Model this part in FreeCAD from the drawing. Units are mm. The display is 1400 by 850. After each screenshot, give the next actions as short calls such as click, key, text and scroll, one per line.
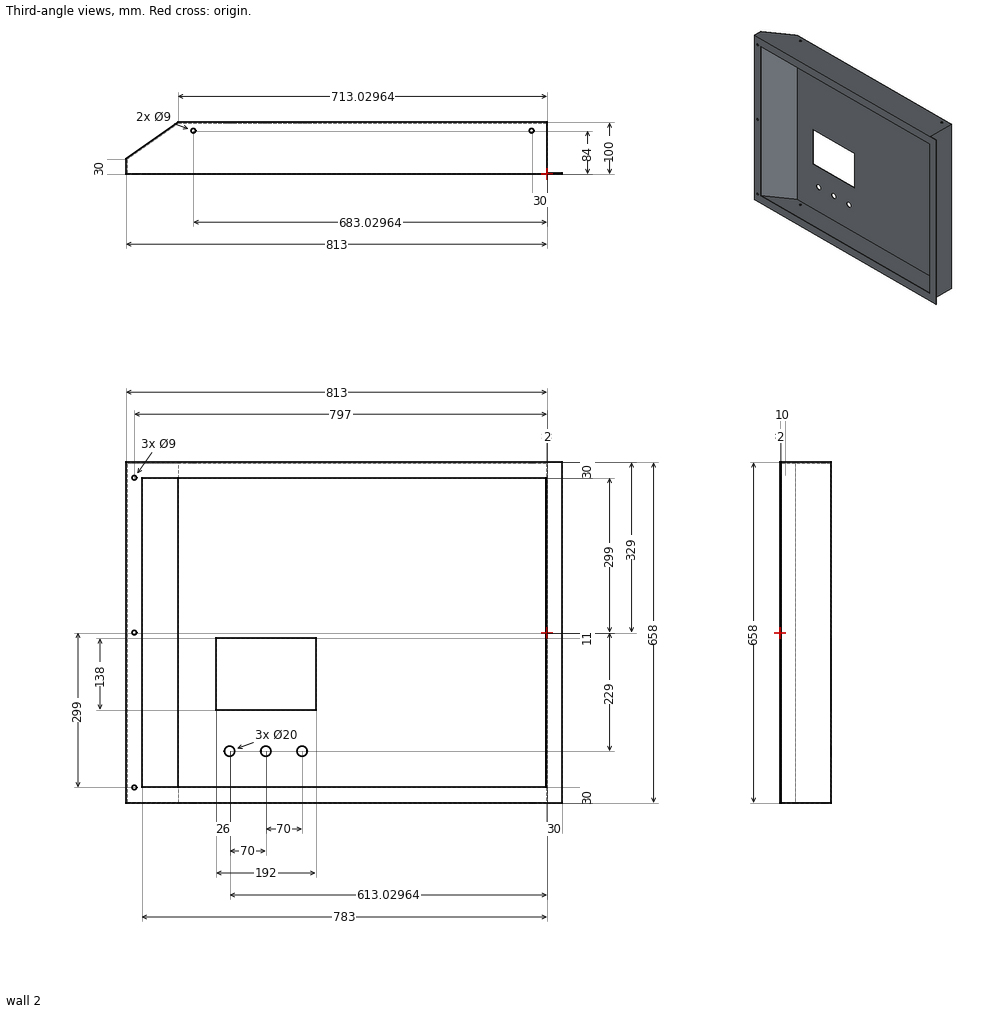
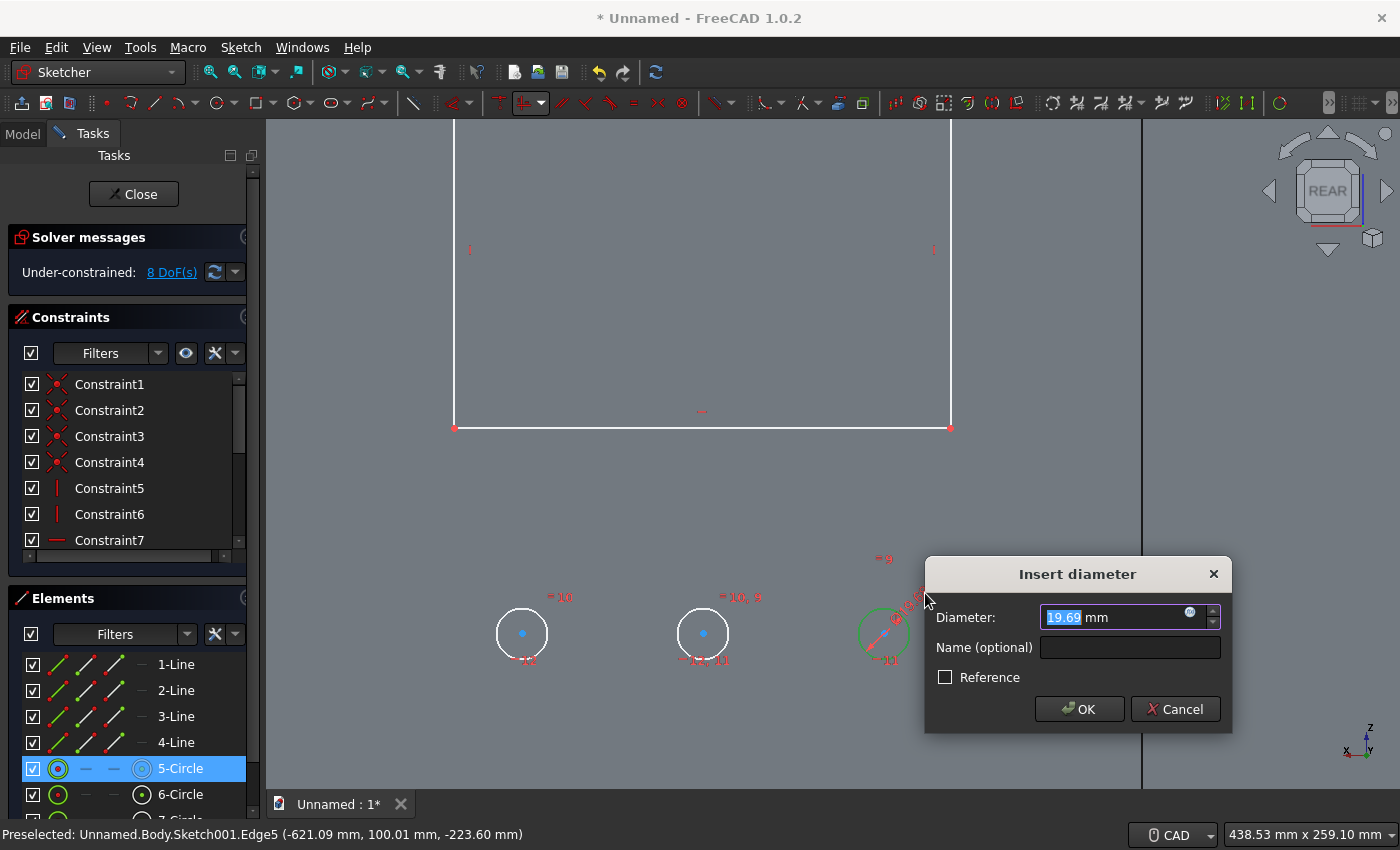
text(20)
key(Return)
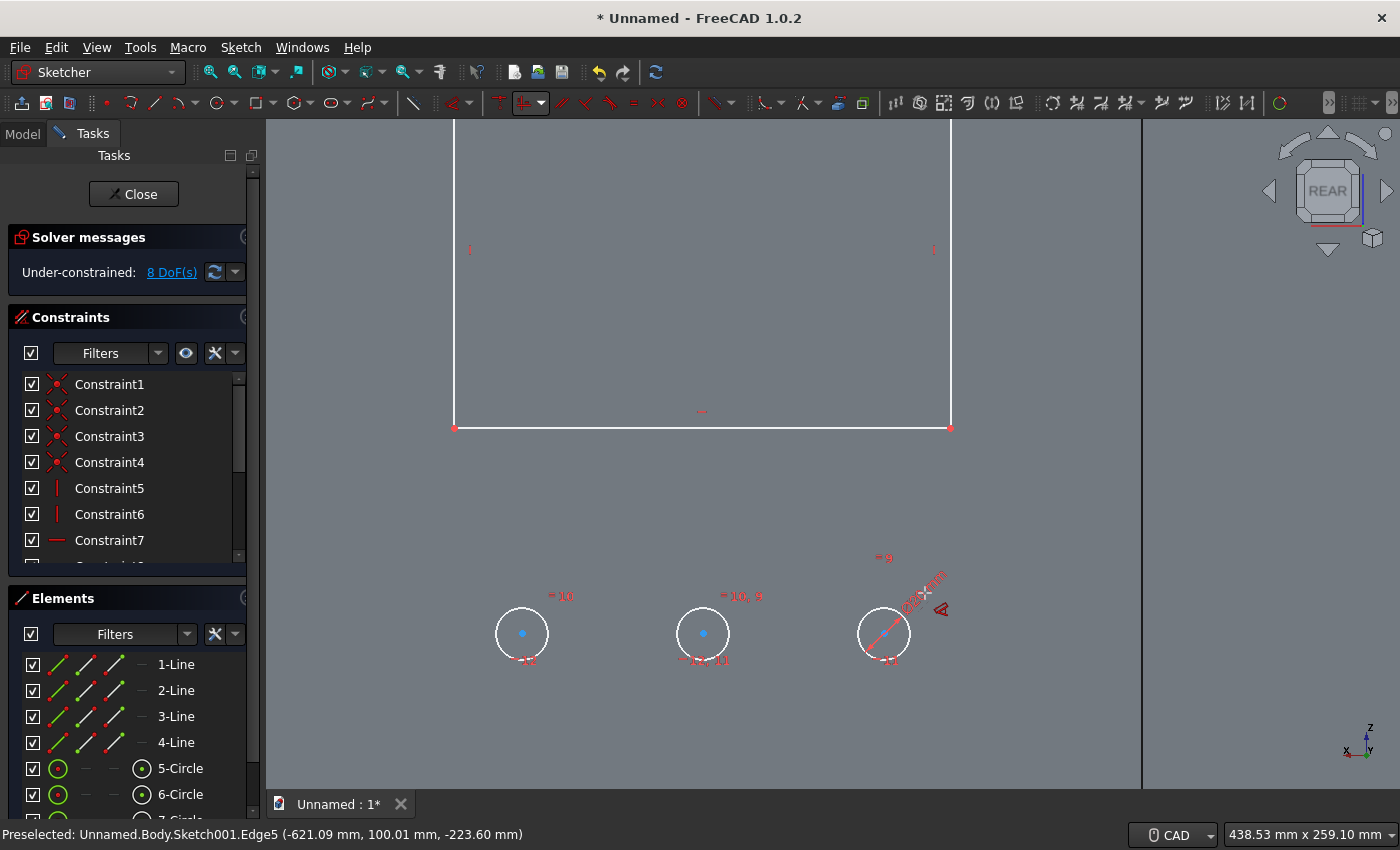
click(454, 178)
click(420, 288)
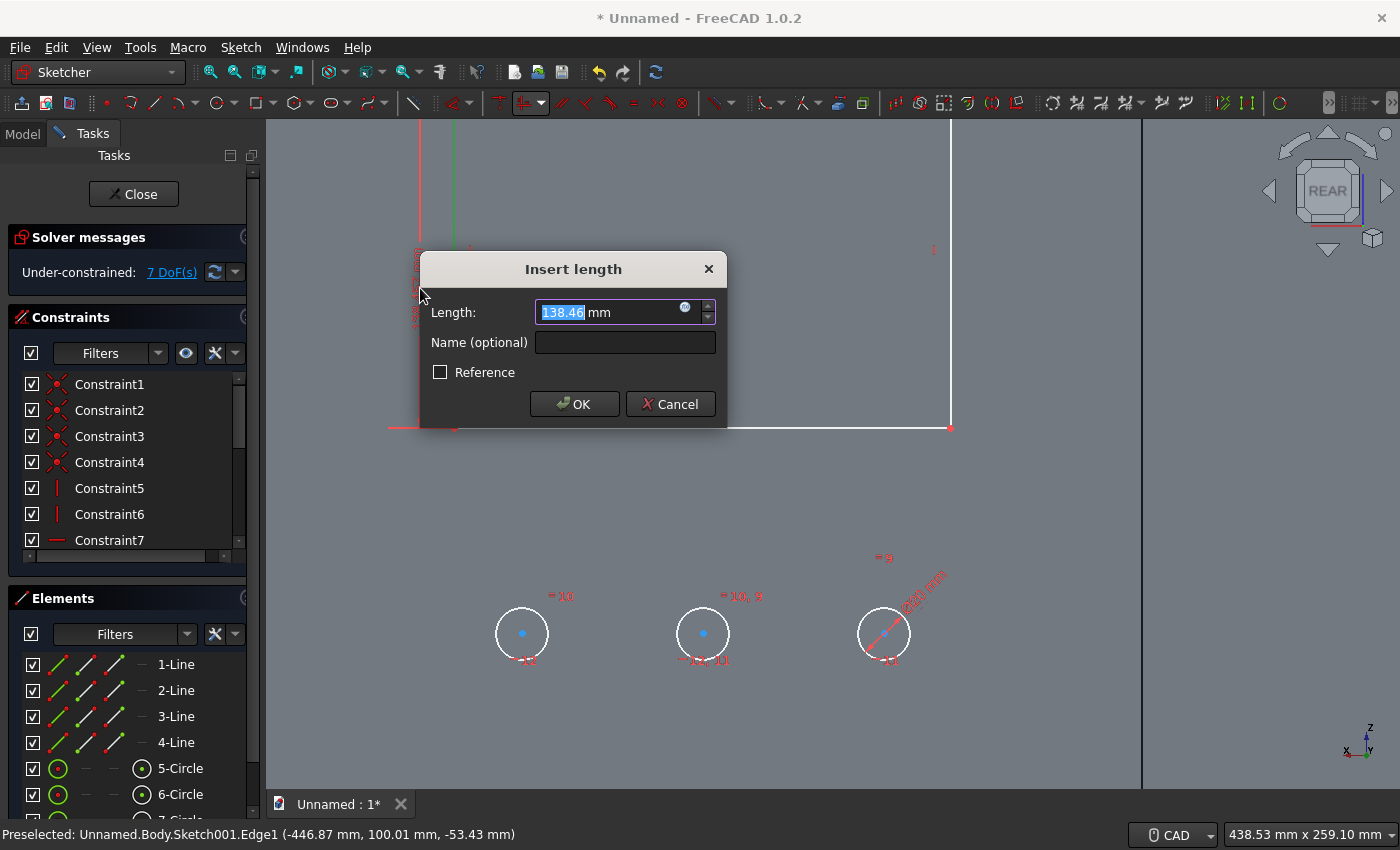
text(138)
key(Return)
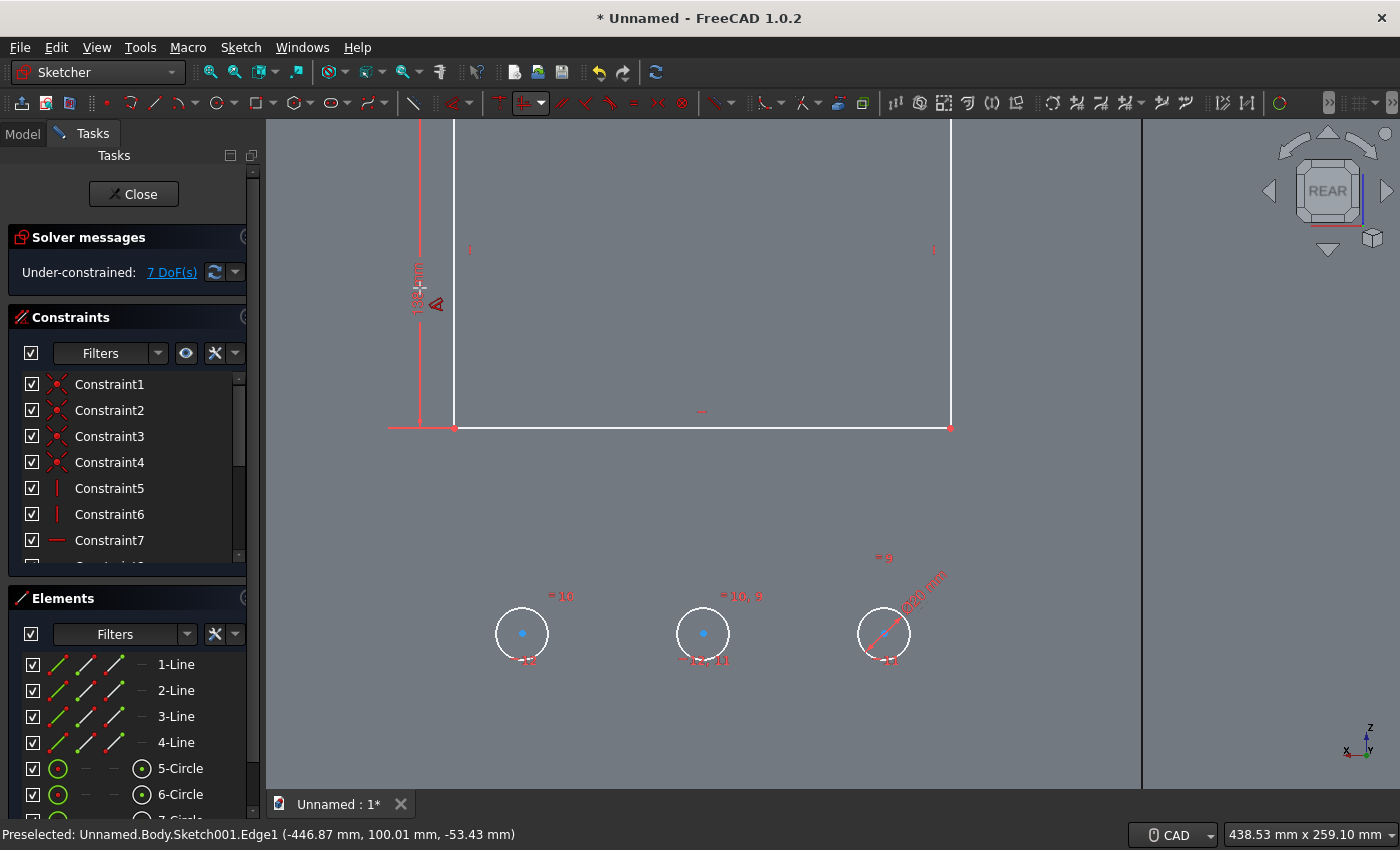
click(603, 428)
click(702, 462)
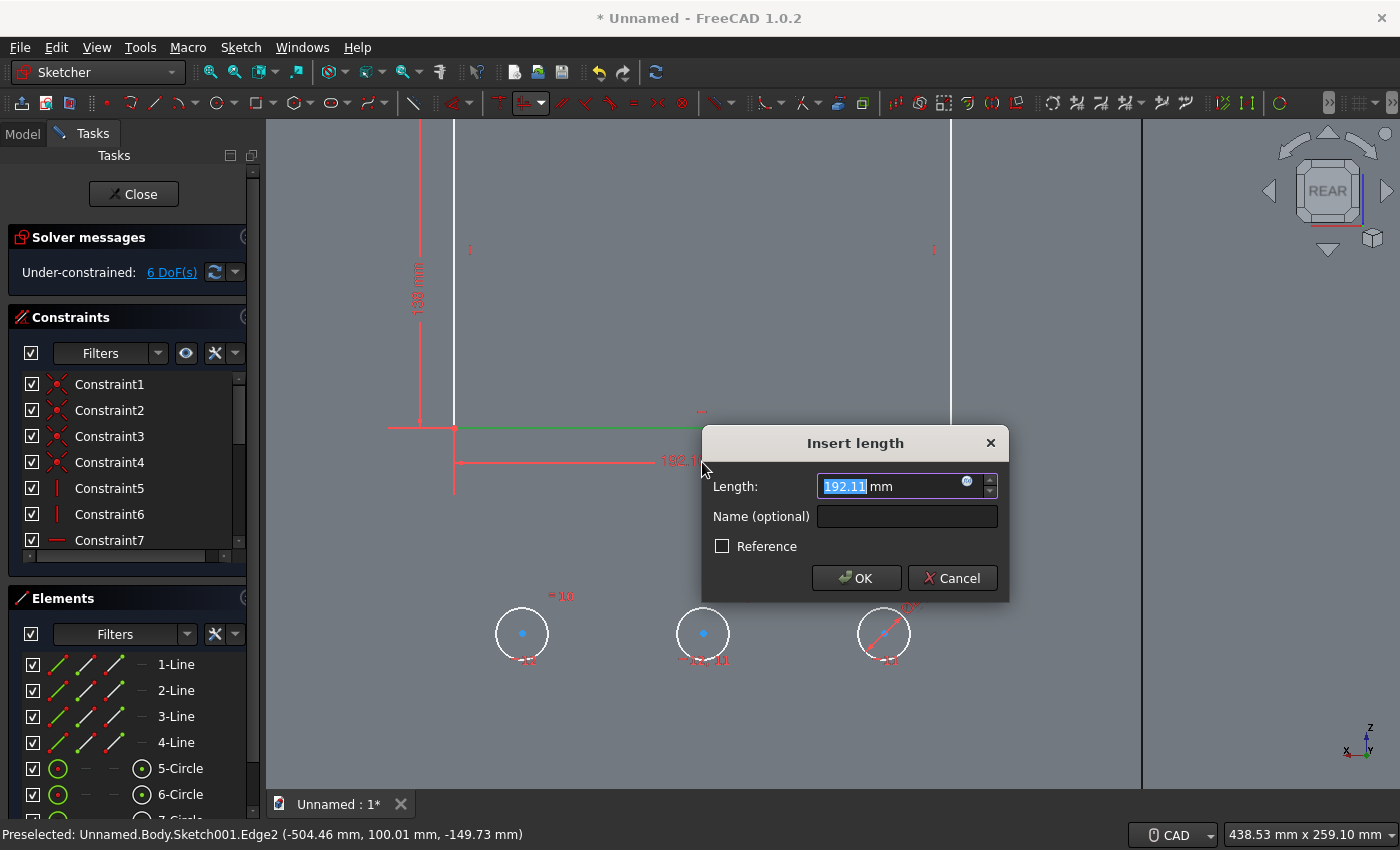
text(192)
key(Return)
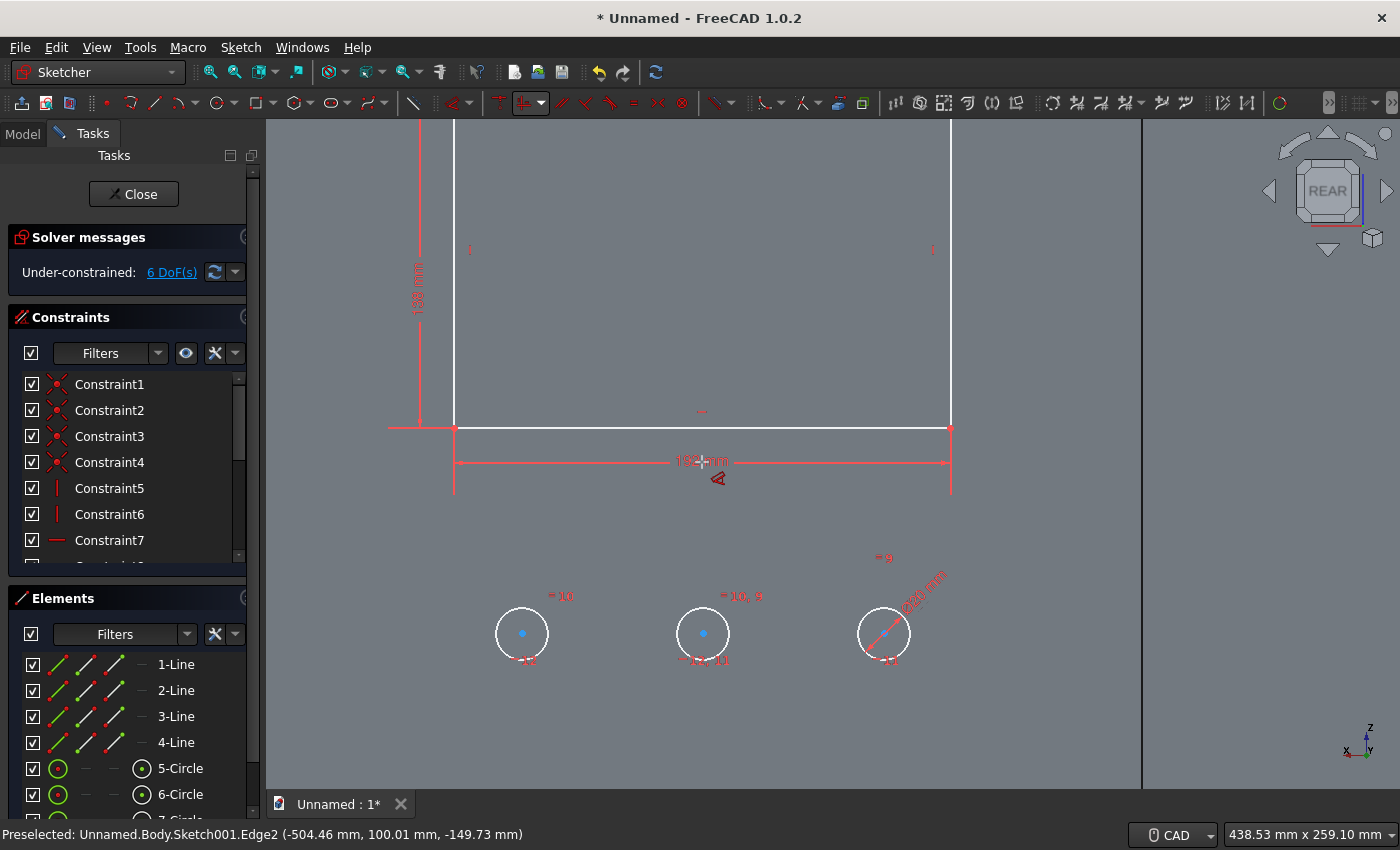
scroll(890, 637, down, 2)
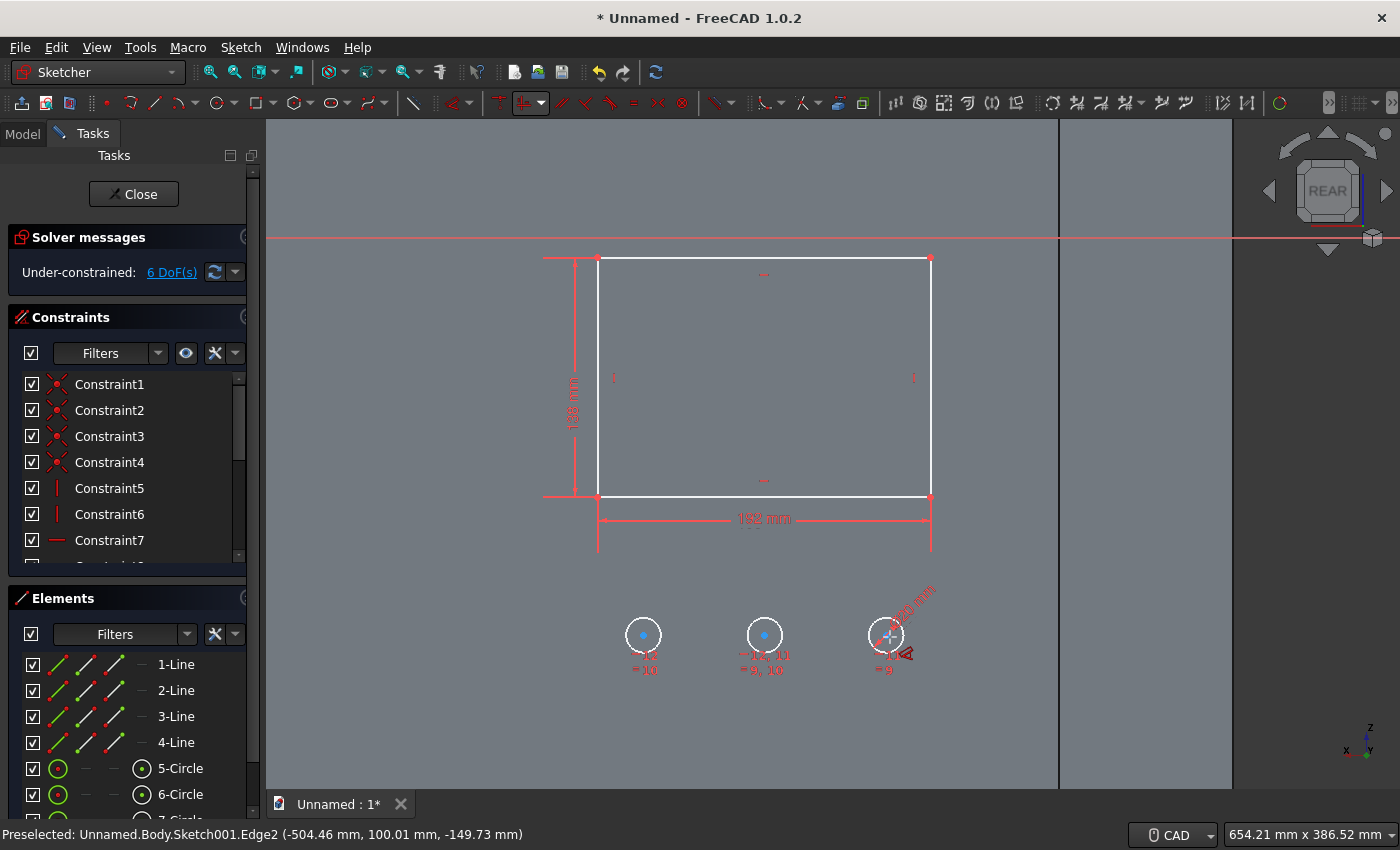
scroll(598, 258, up, 4)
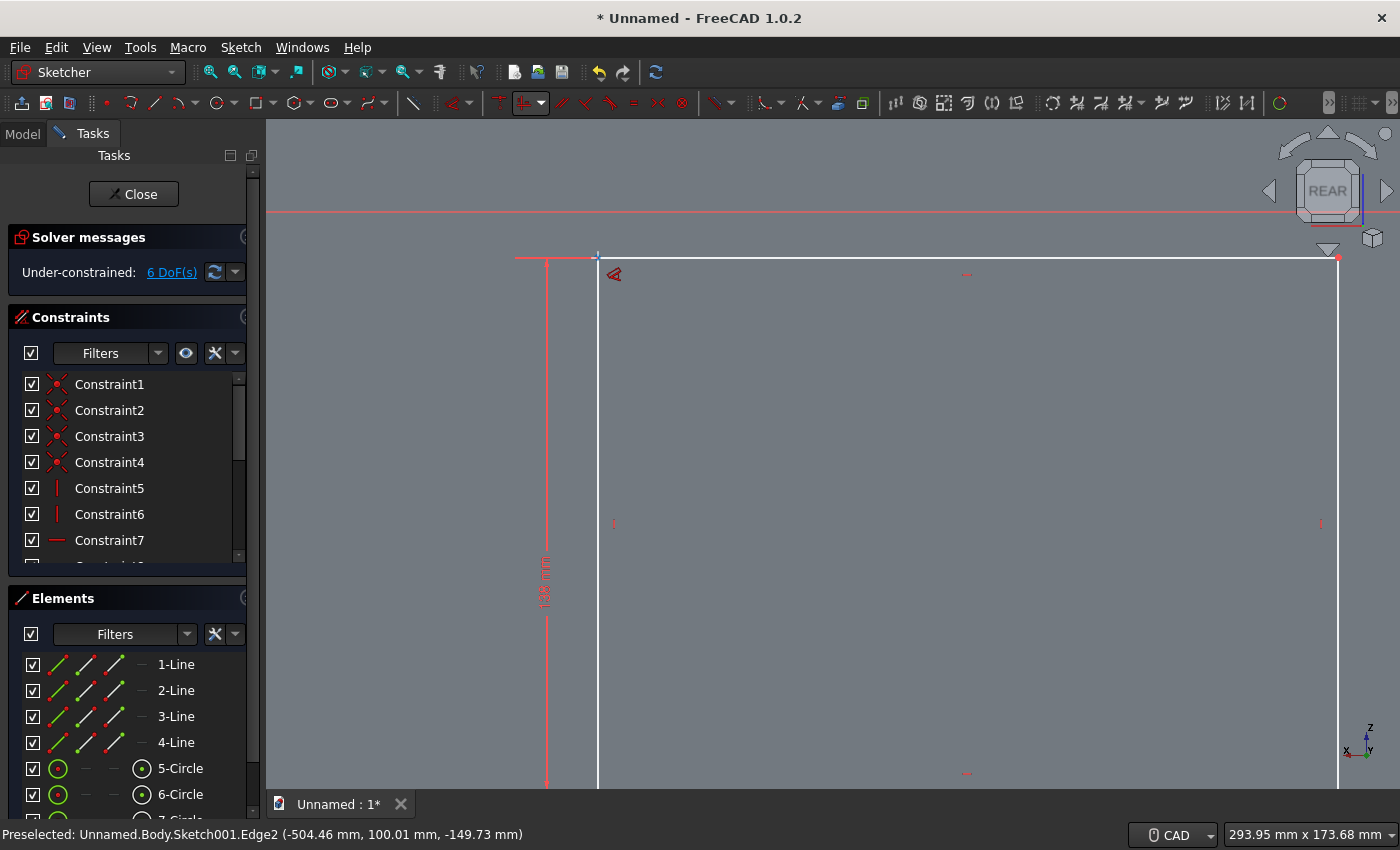
click(598, 258)
click(632, 235)